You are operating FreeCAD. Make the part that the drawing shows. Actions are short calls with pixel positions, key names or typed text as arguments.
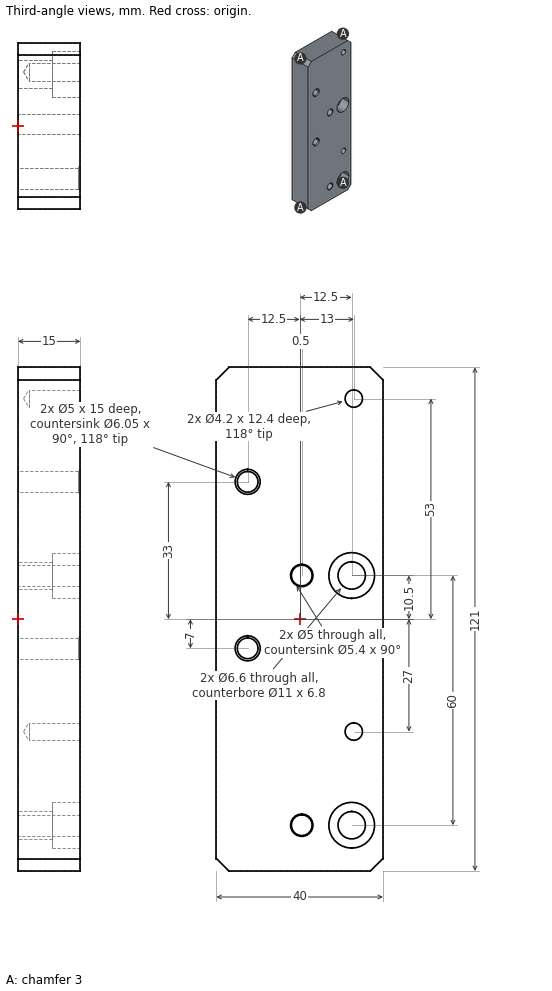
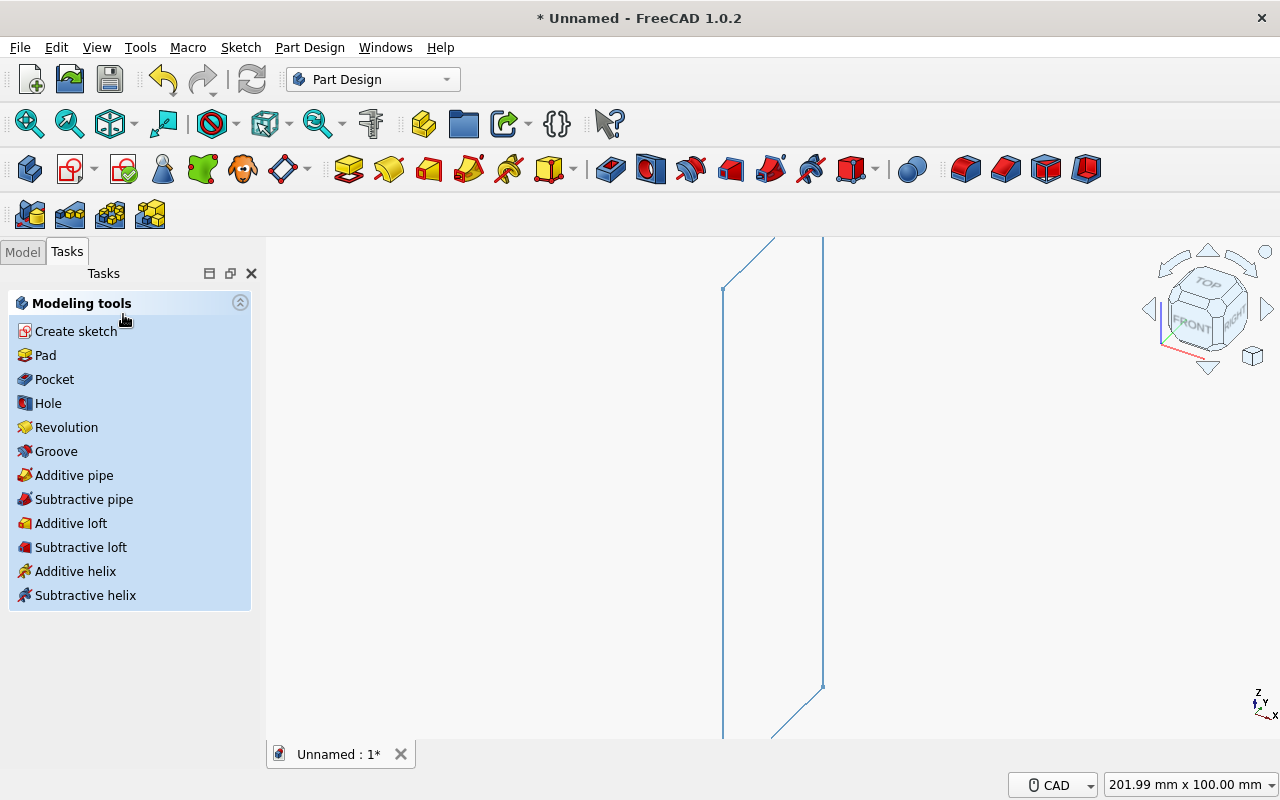
click(350, 170)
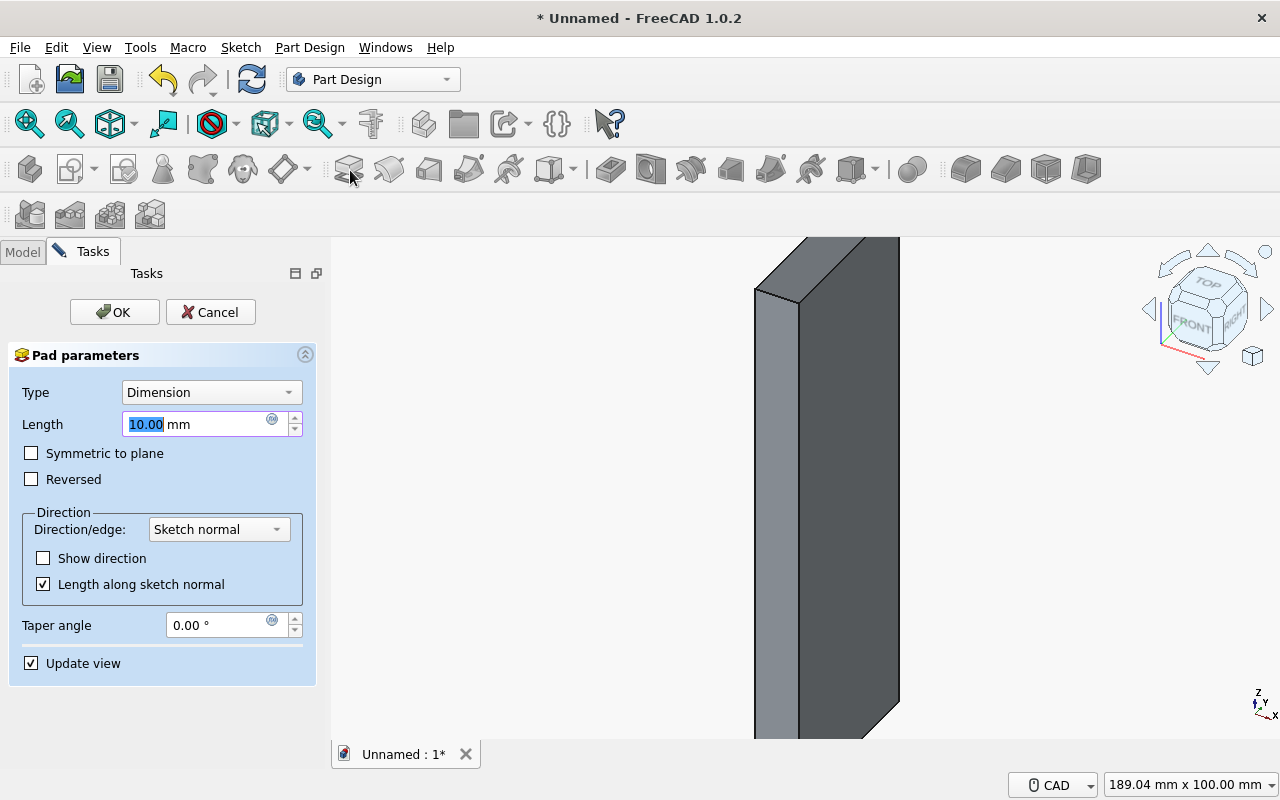
text(15)
key(Tab)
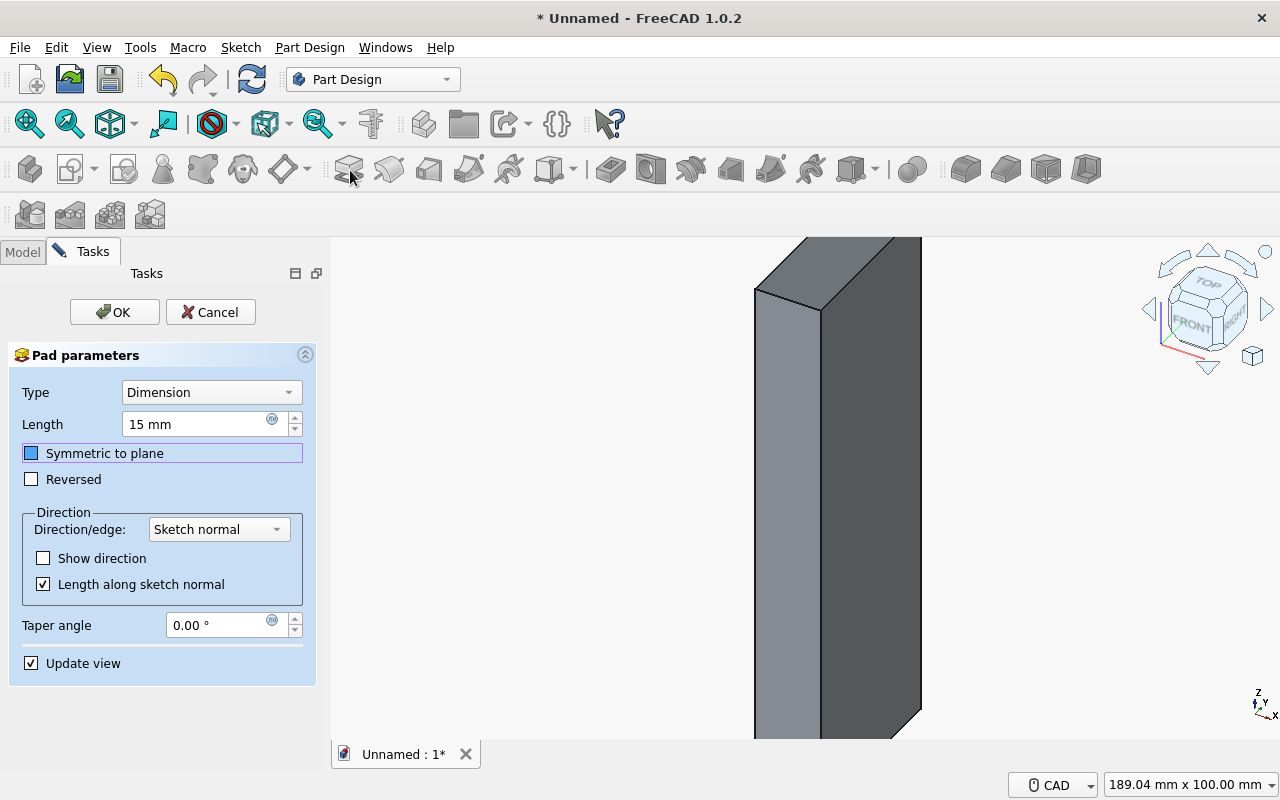
click(115, 312)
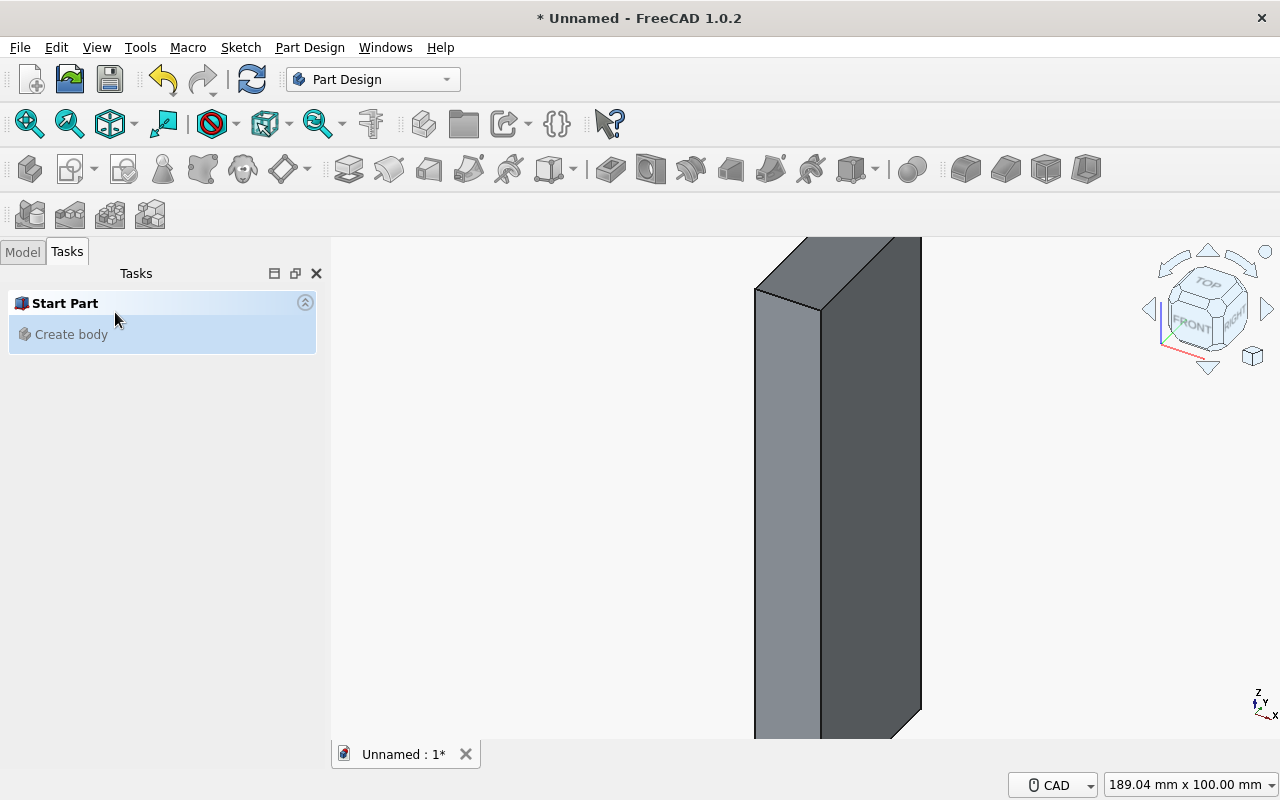
click(30, 124)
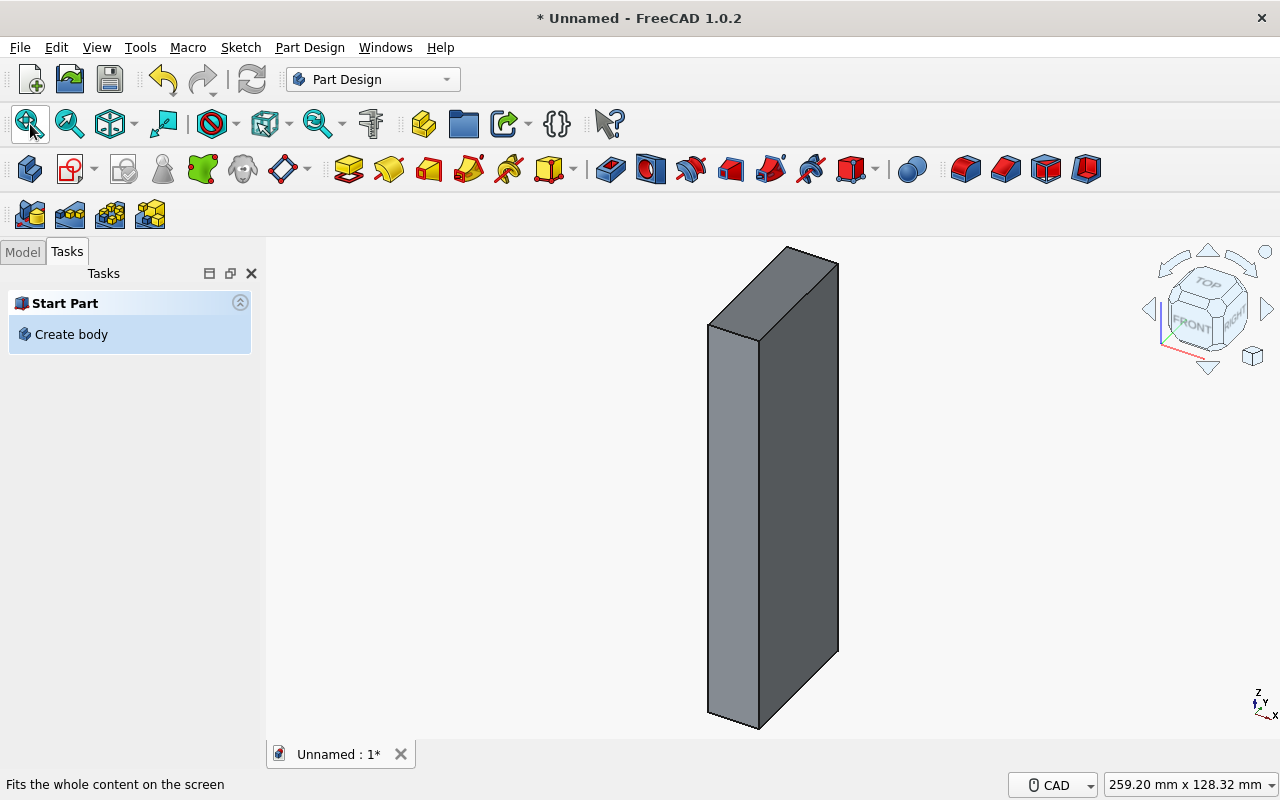
click(798, 606)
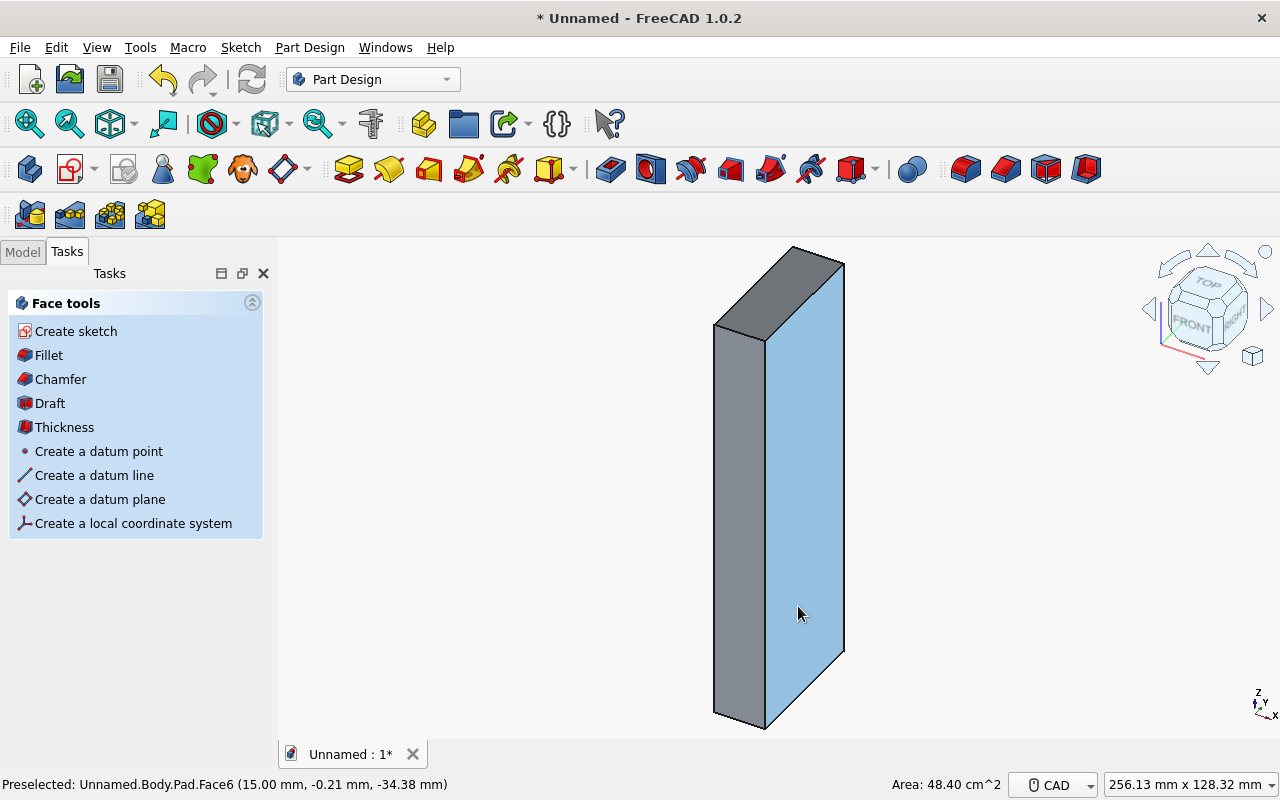
click(70, 170)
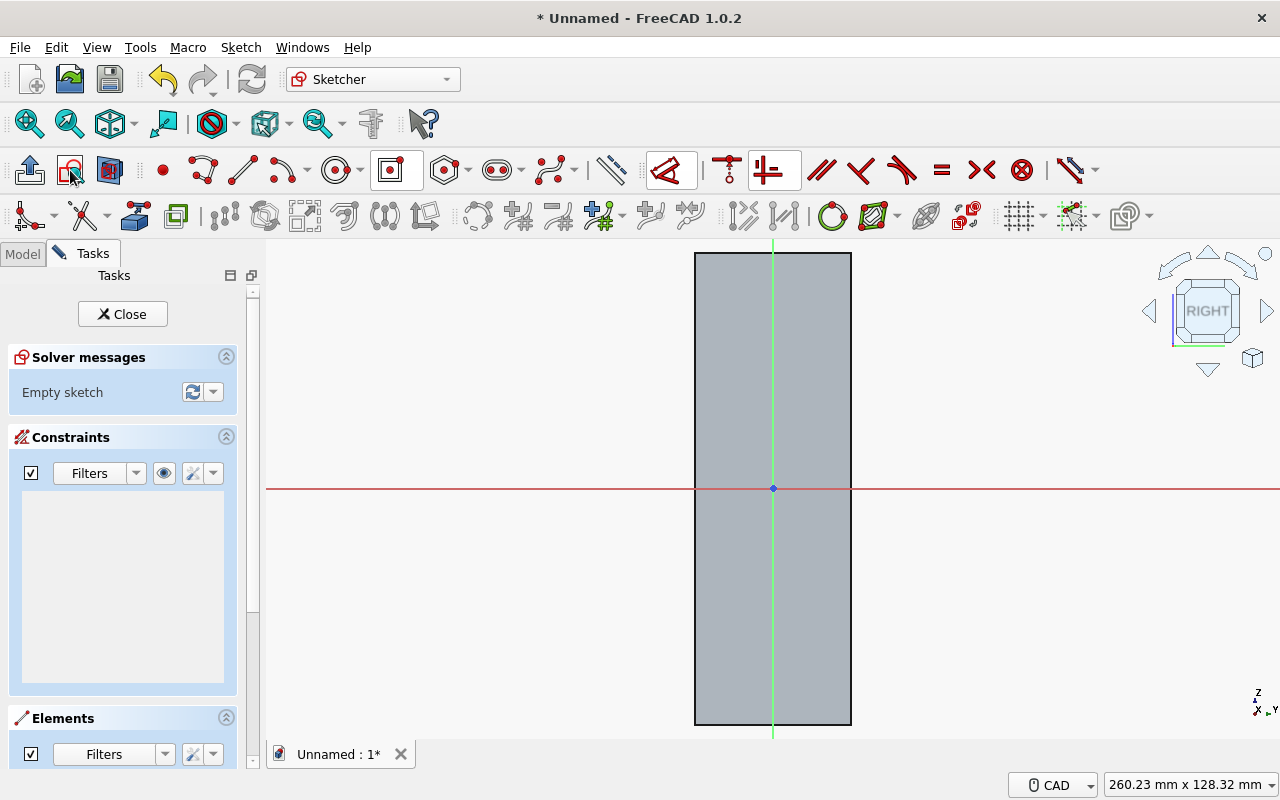
scroll(294, 711, down, 1)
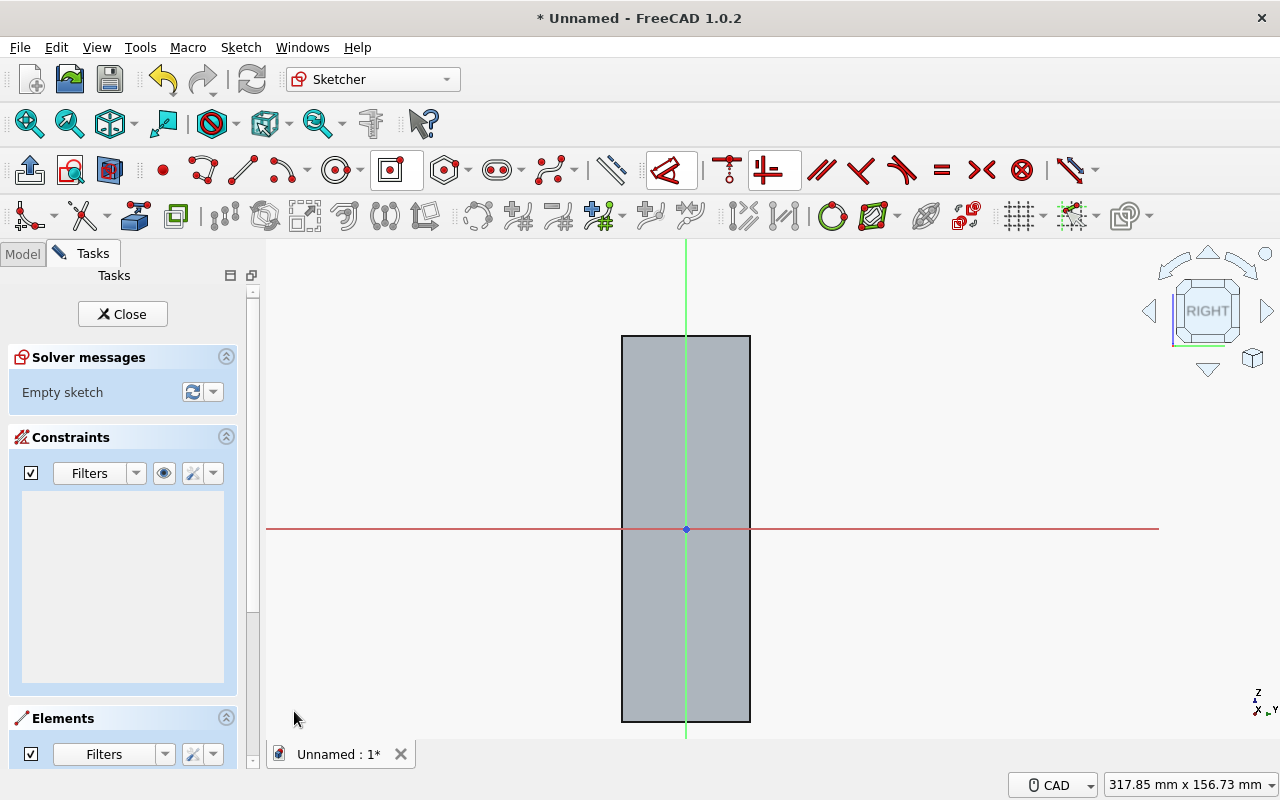
click(336, 170)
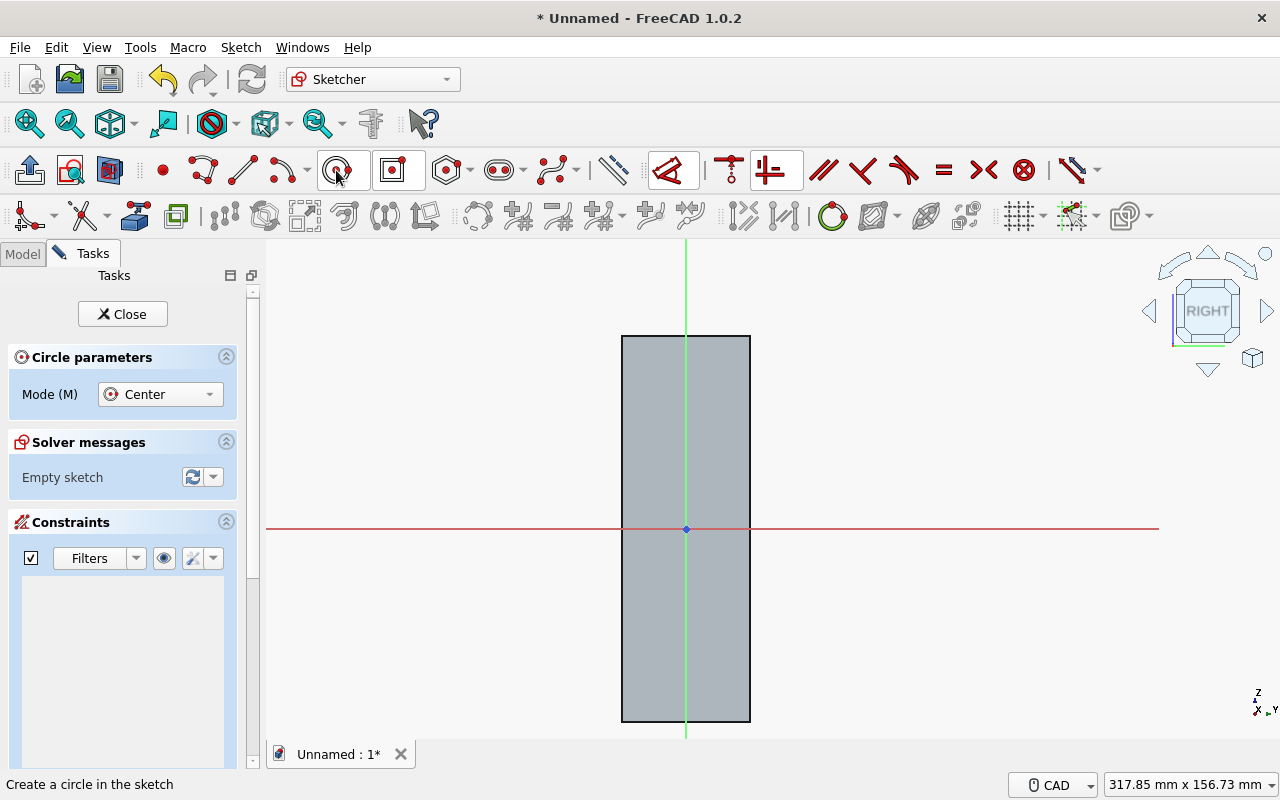
scroll(728, 360, up, 7)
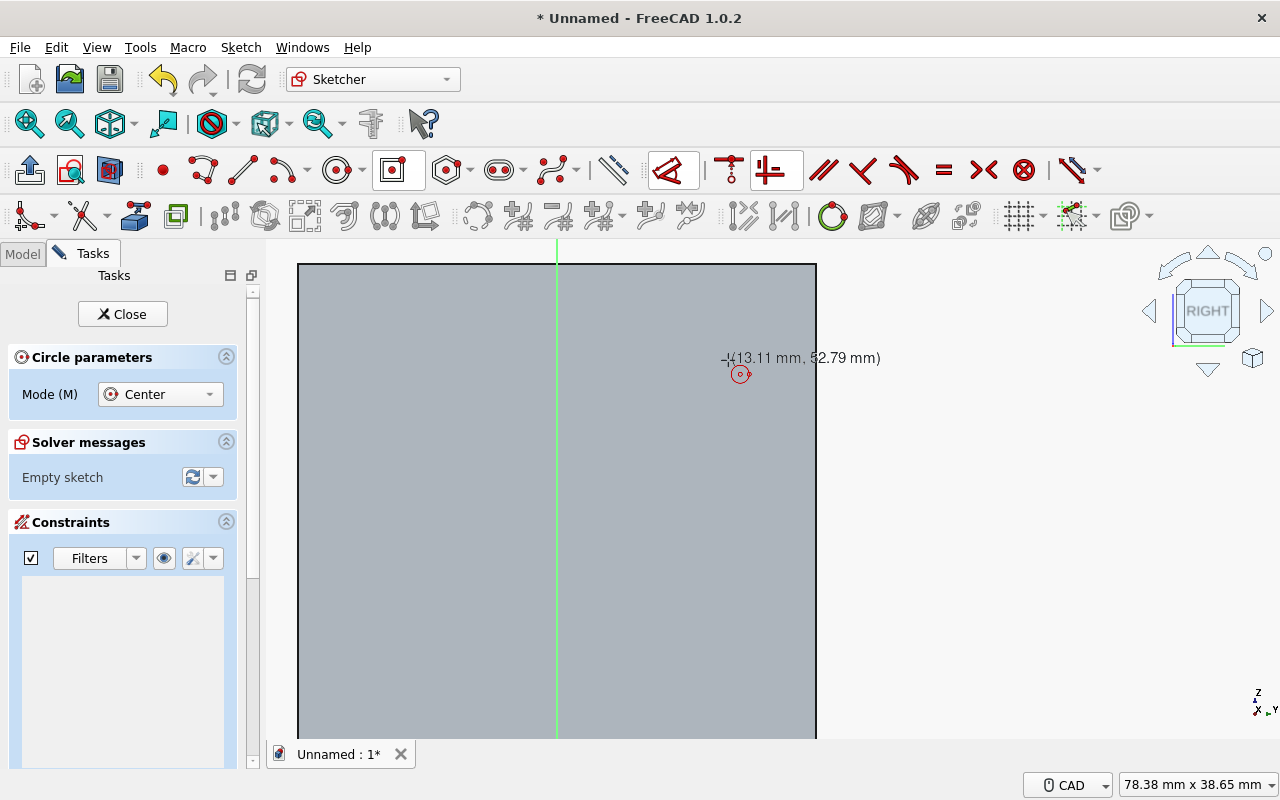
scroll(726, 321, down, 6)